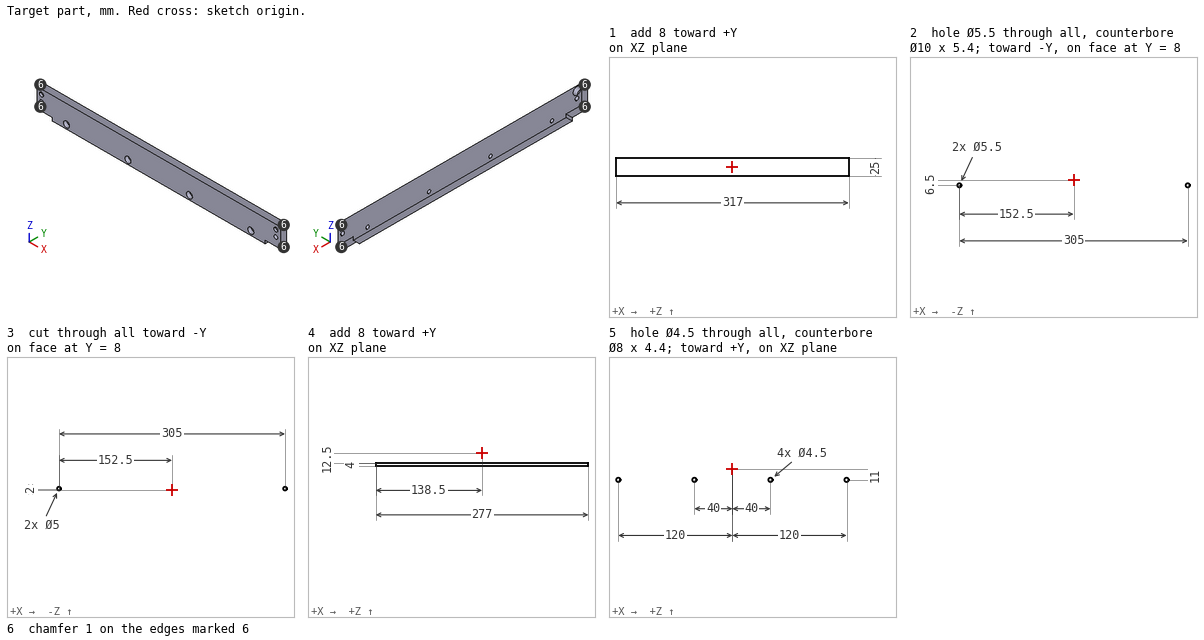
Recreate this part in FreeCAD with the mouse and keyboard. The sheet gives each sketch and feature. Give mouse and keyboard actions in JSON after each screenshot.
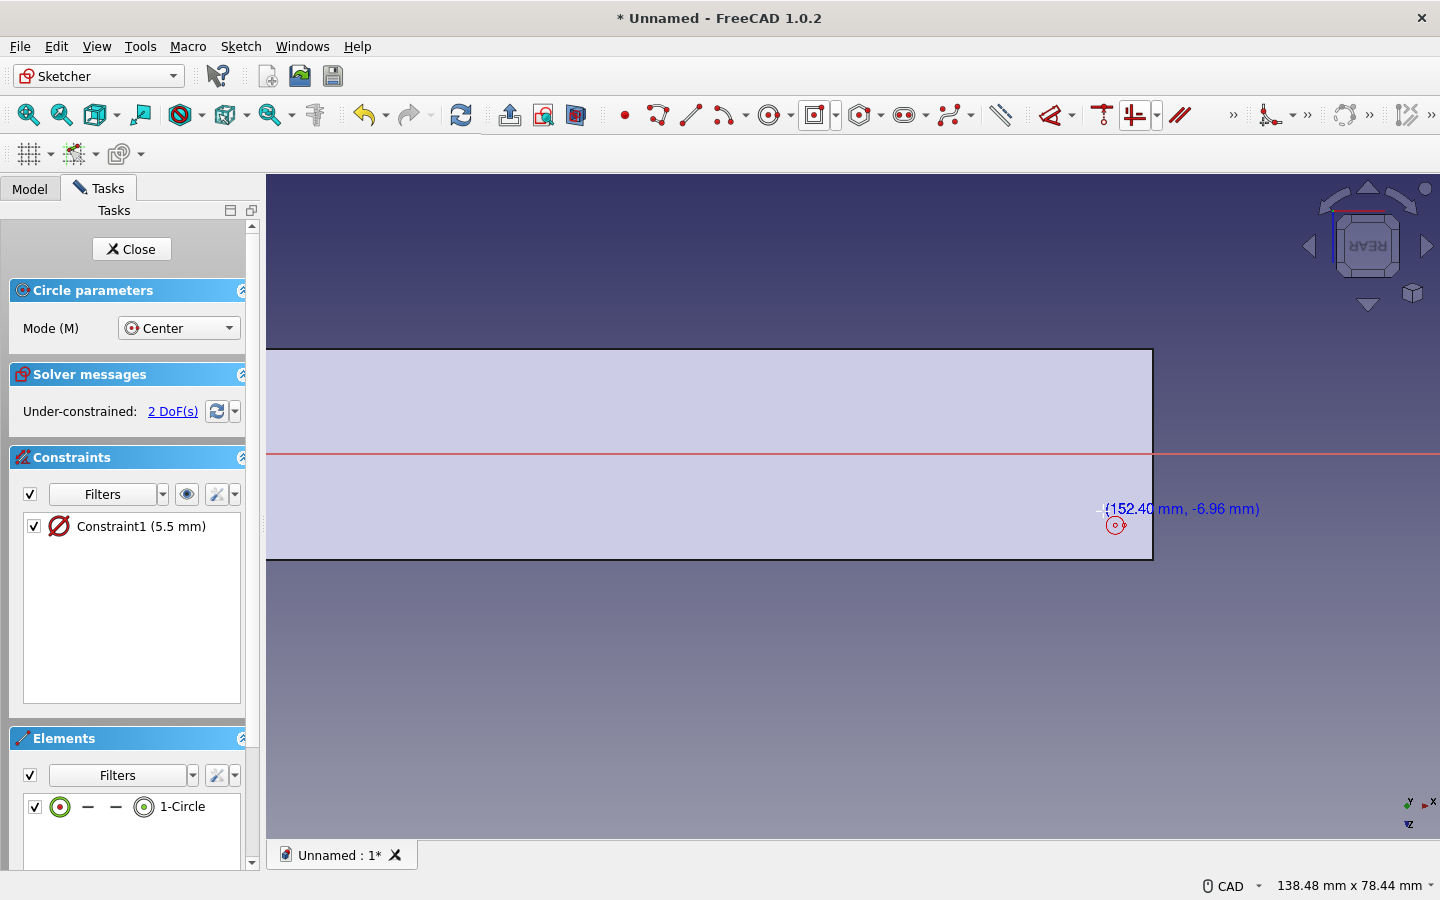
{"action": "scroll", "coordinate": [1104, 511], "scroll_direction": "down", "scroll_amount": 7}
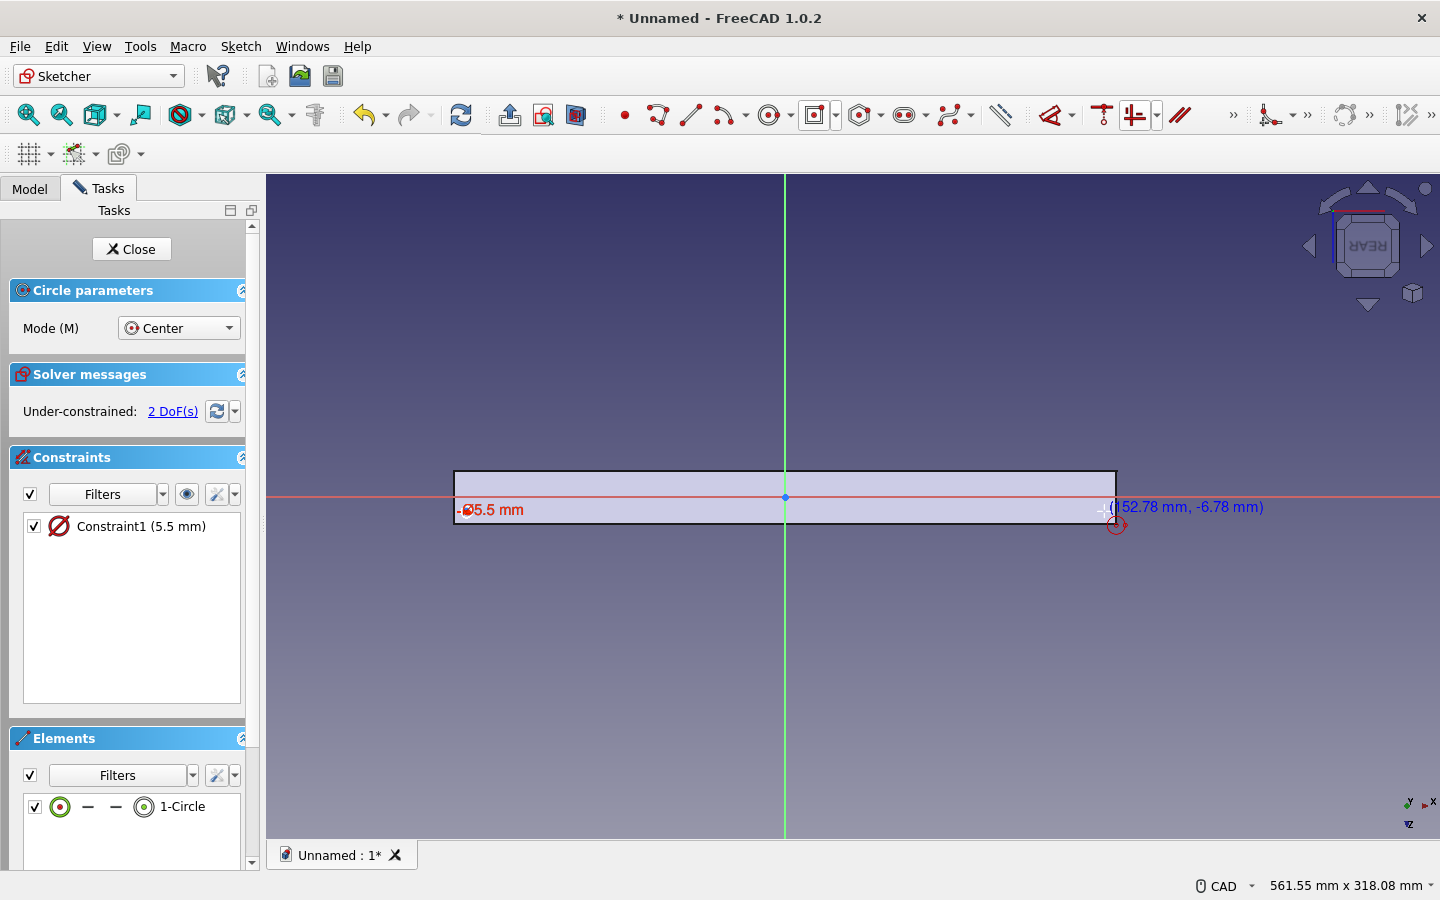
{"action": "left_click", "coordinate": [1104, 511]}
{"action": "mouse_move", "coordinate": [1108, 515]}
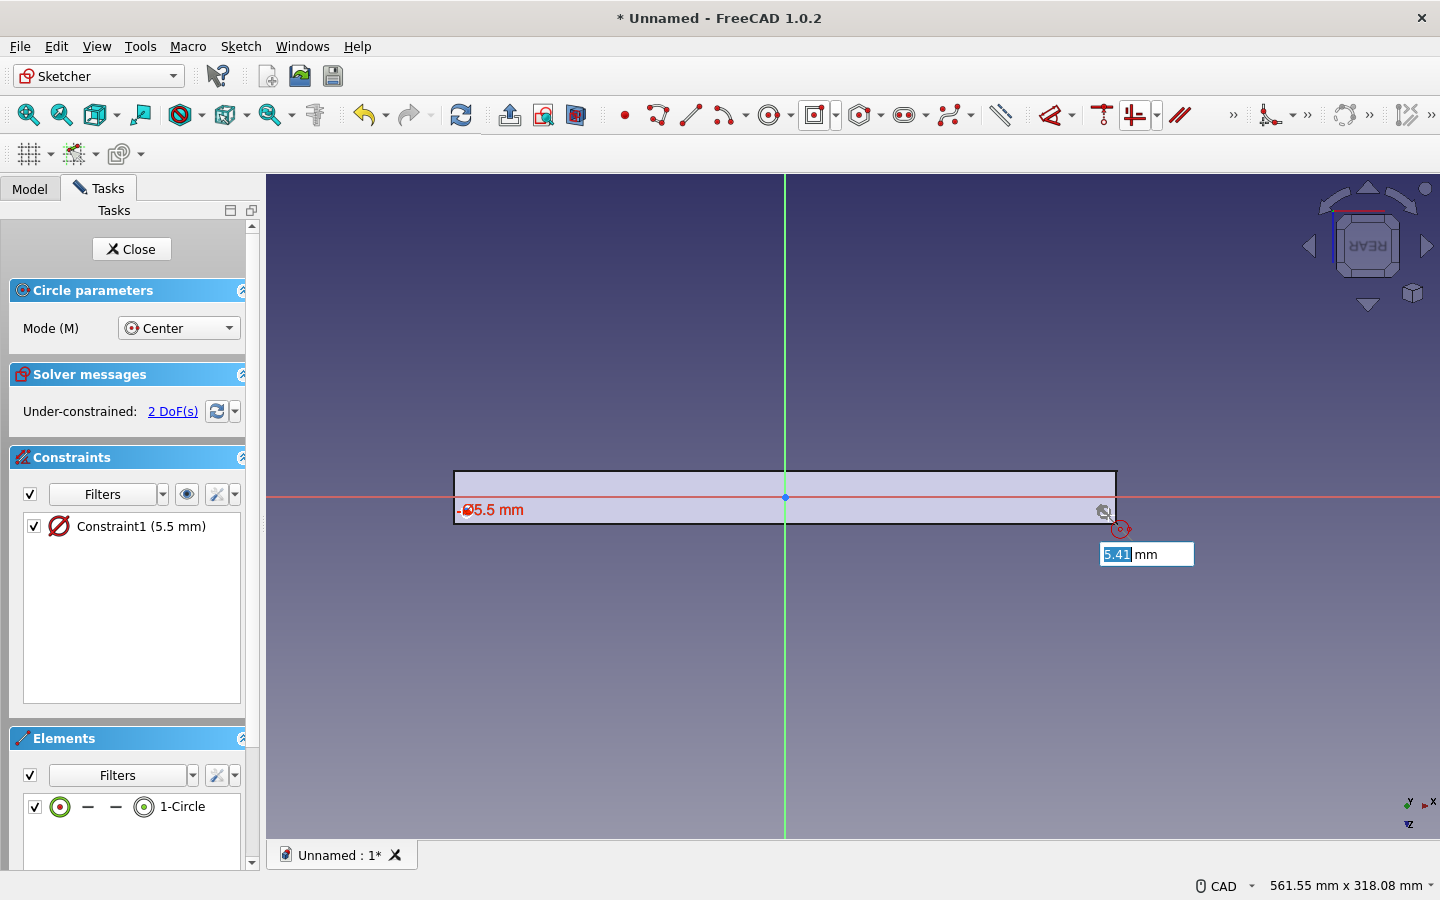
{"action": "type", "text": "5.5"}
{"action": "key", "text": "Return"}
{"action": "key", "text": "Escape"}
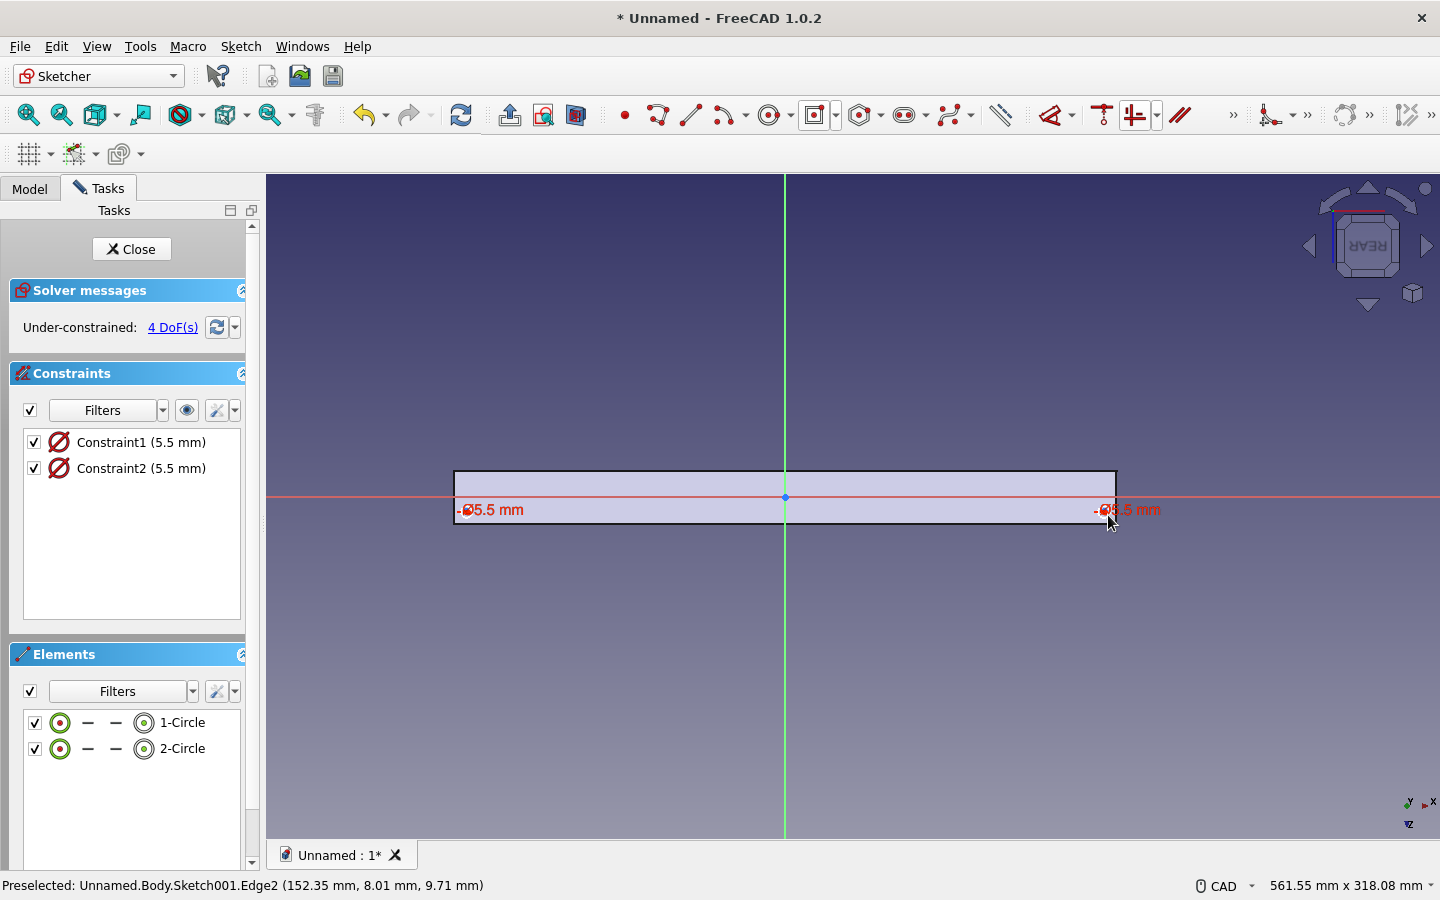
{"action": "left_click", "coordinate": [467, 512]}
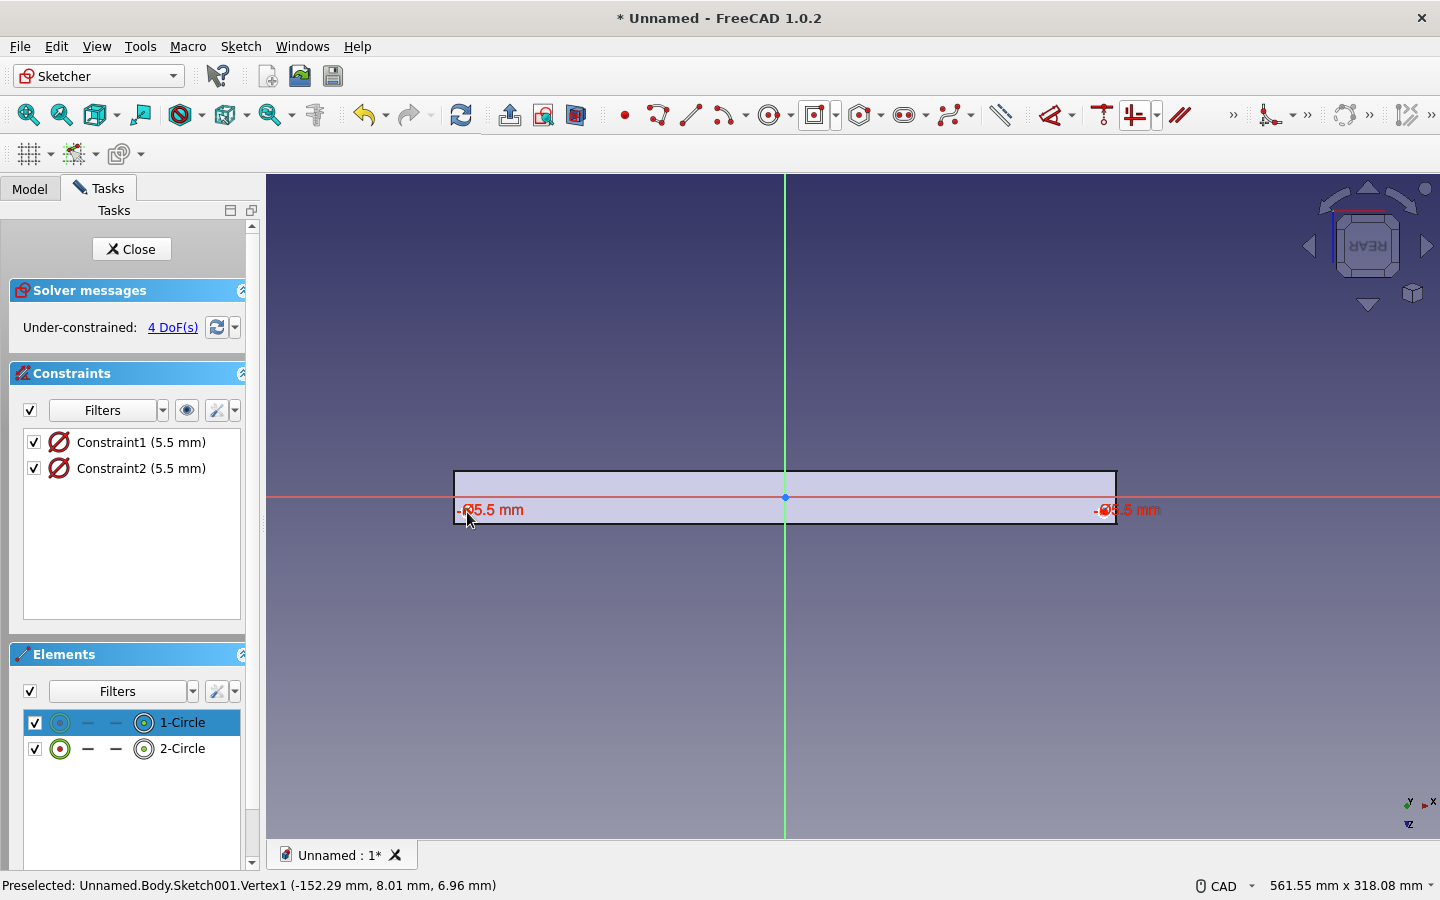
{"action": "left_click", "coordinate": [1104, 512]}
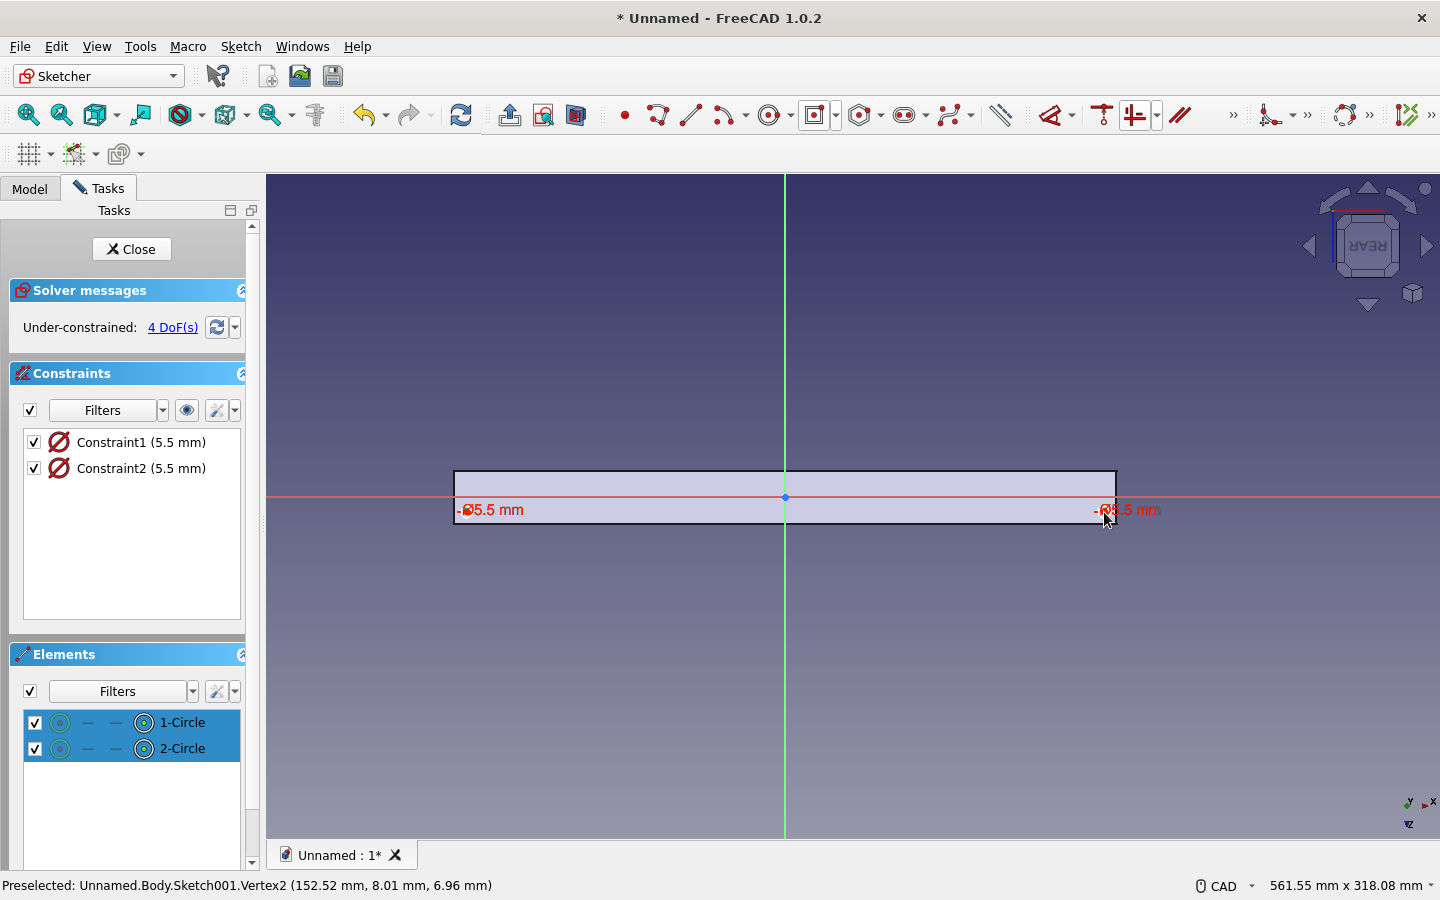
{"action": "left_click", "coordinate": [1156, 116]}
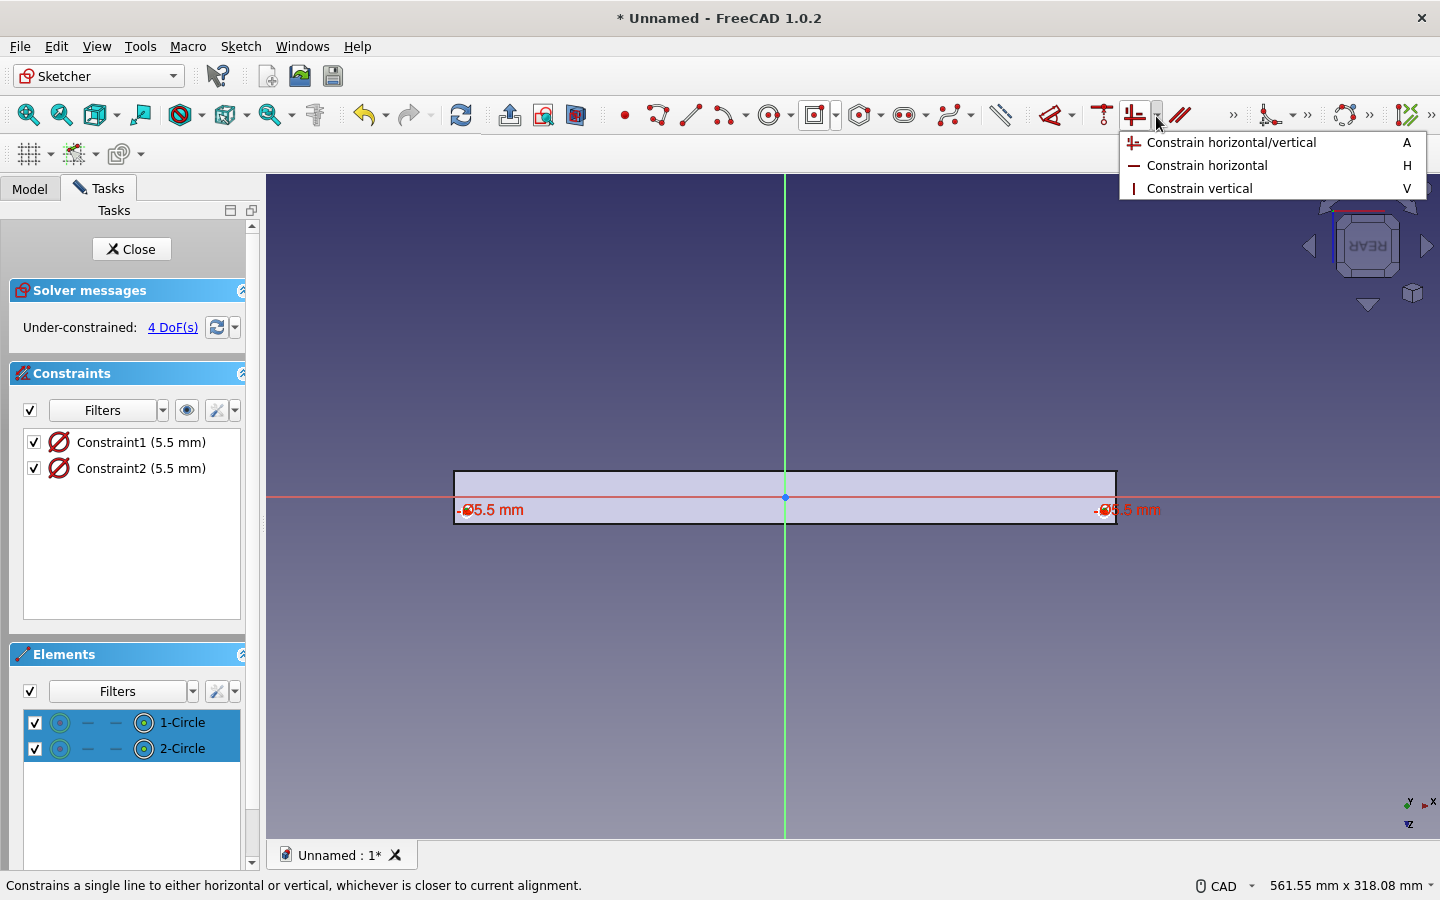
{"action": "left_click", "coordinate": [1273, 166]}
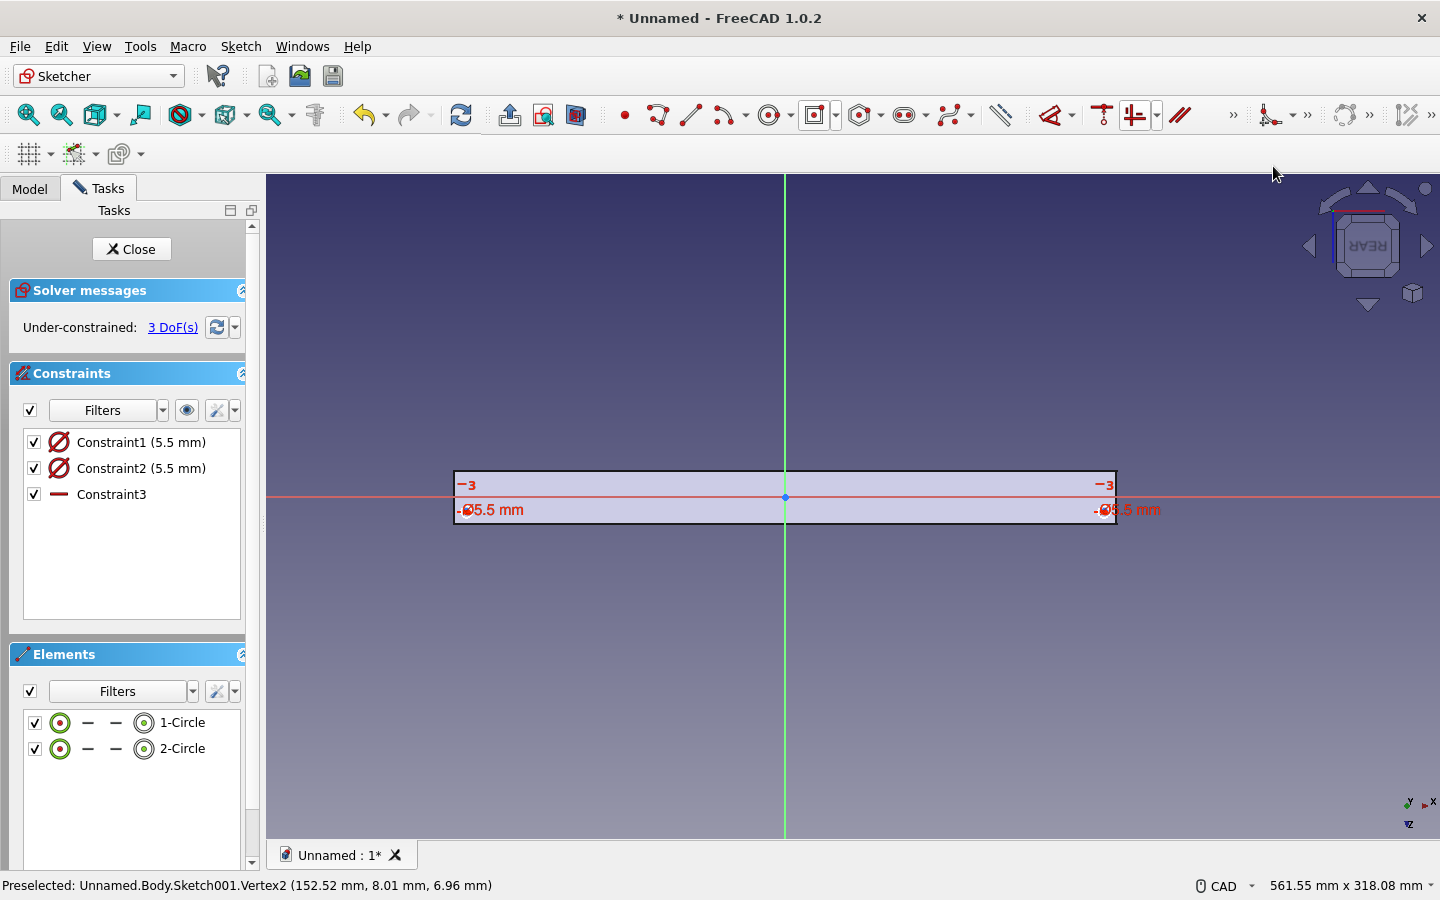
{"action": "left_click", "coordinate": [1050, 116]}